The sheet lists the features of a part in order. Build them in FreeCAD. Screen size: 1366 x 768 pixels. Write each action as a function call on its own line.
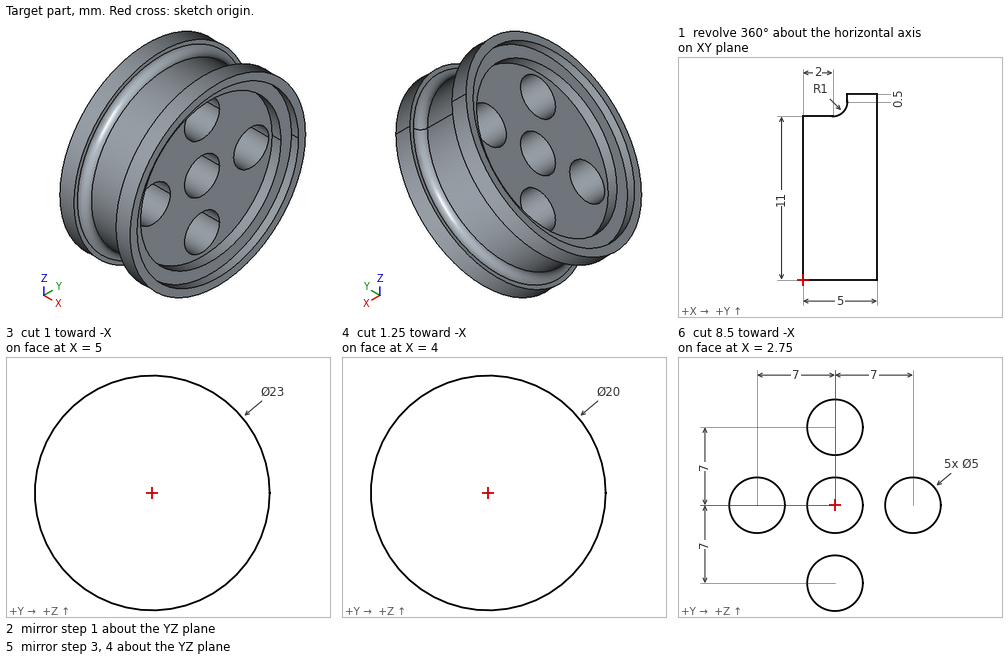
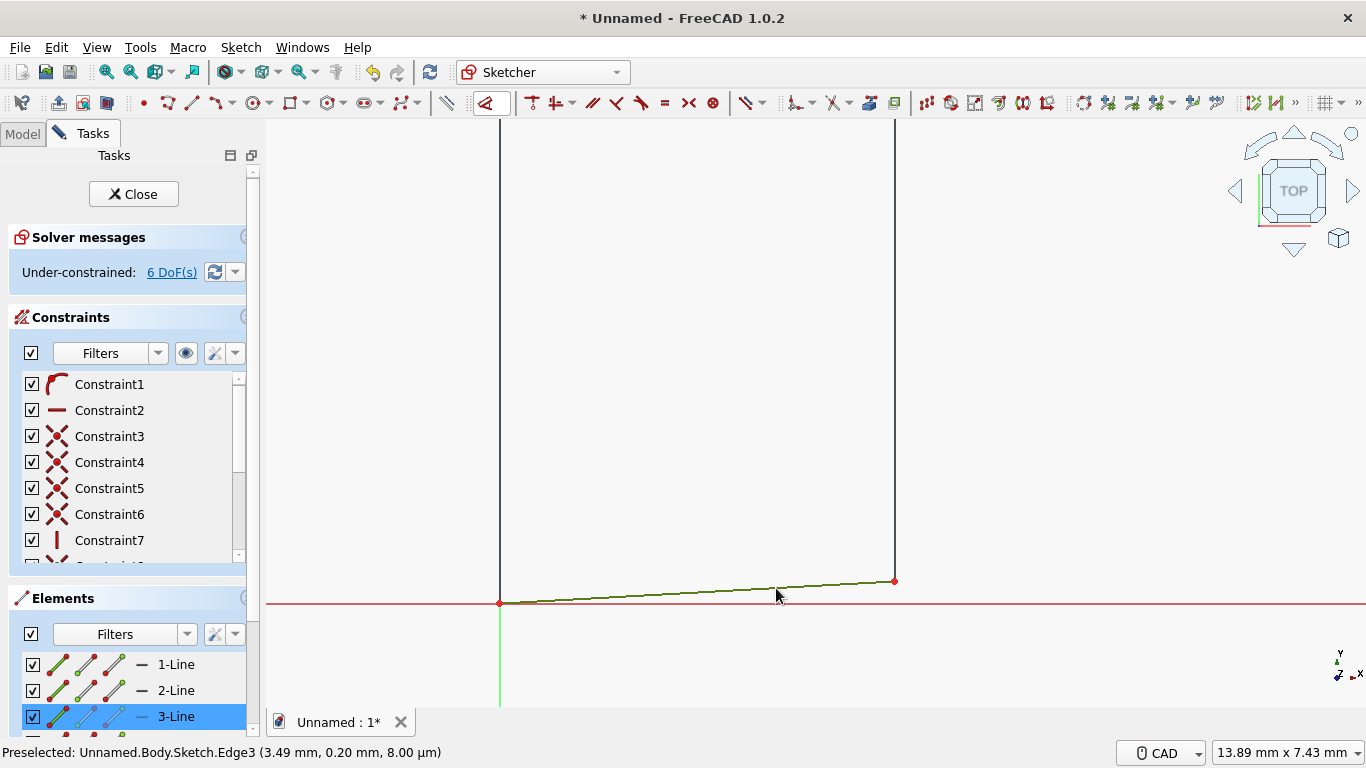
key(h)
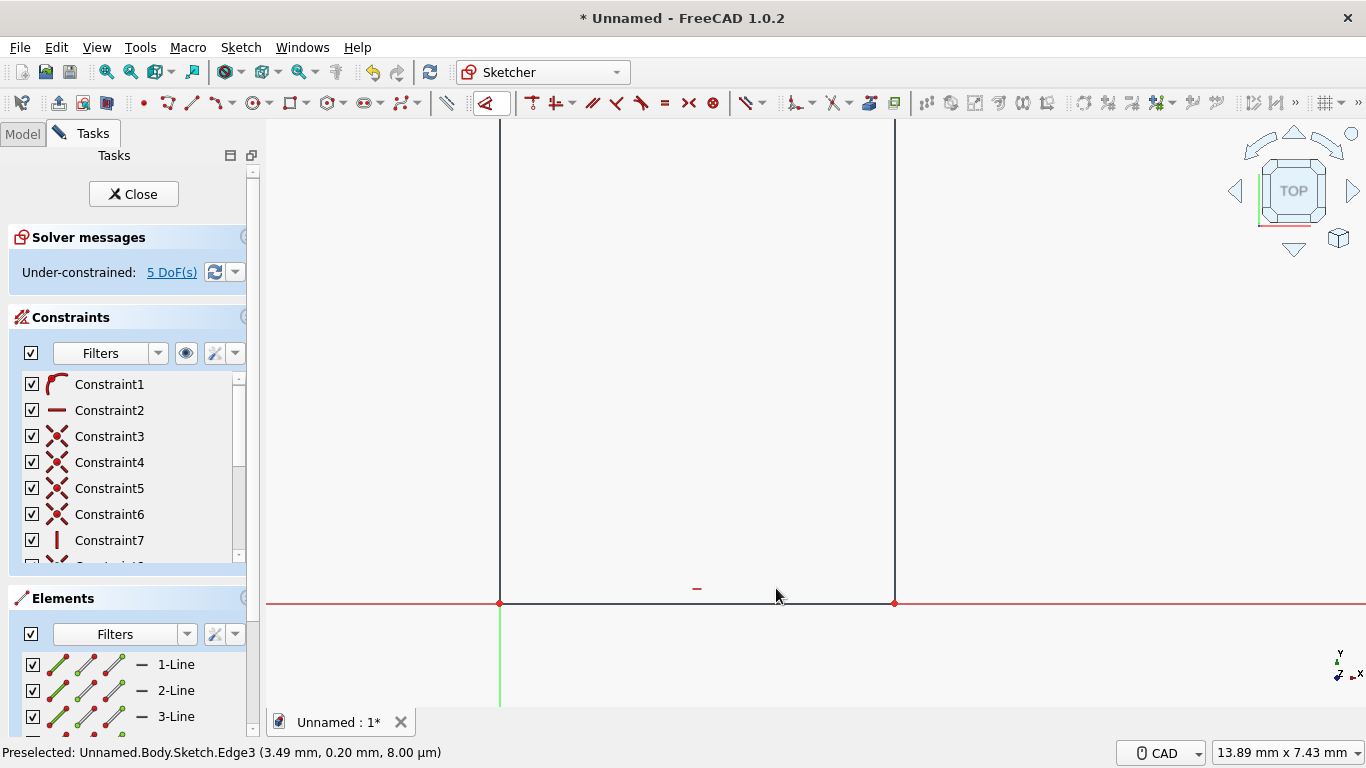
key(d)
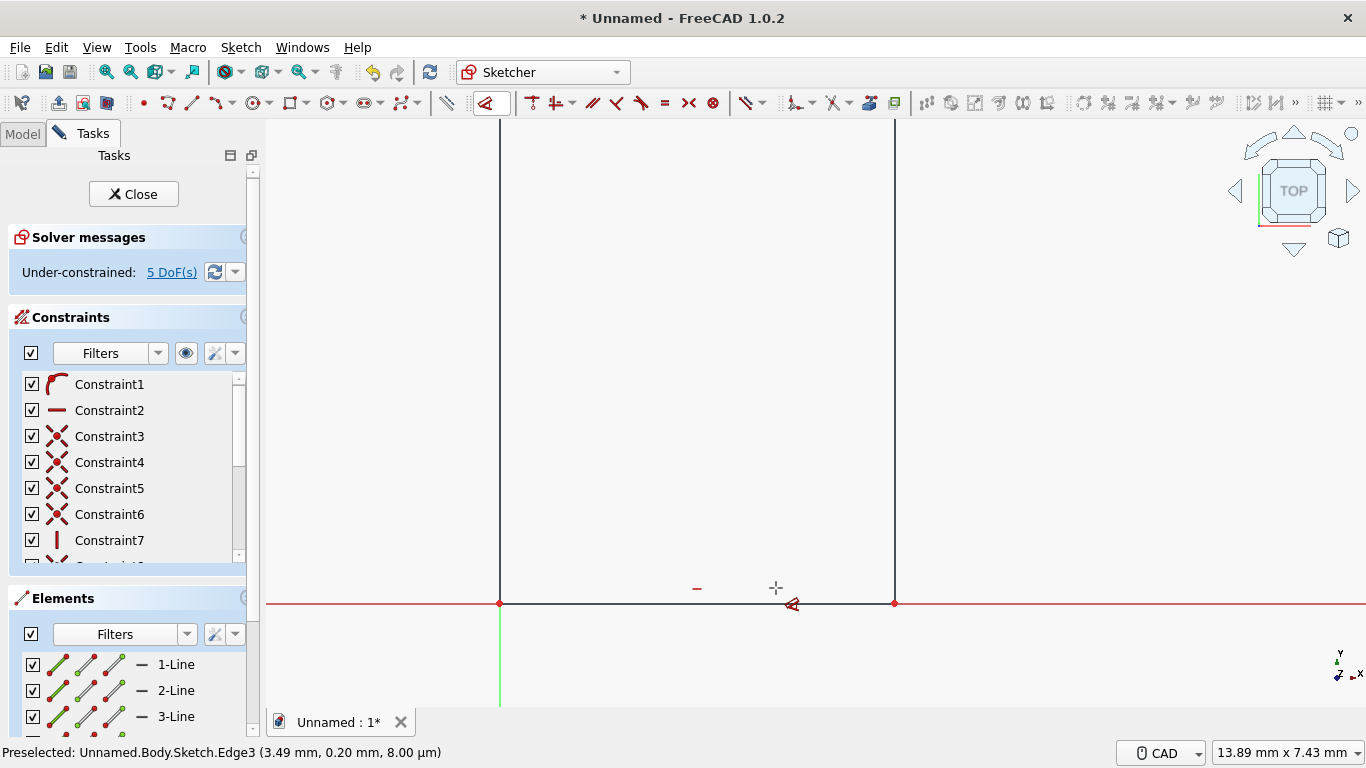
scroll(777, 590, down, 5)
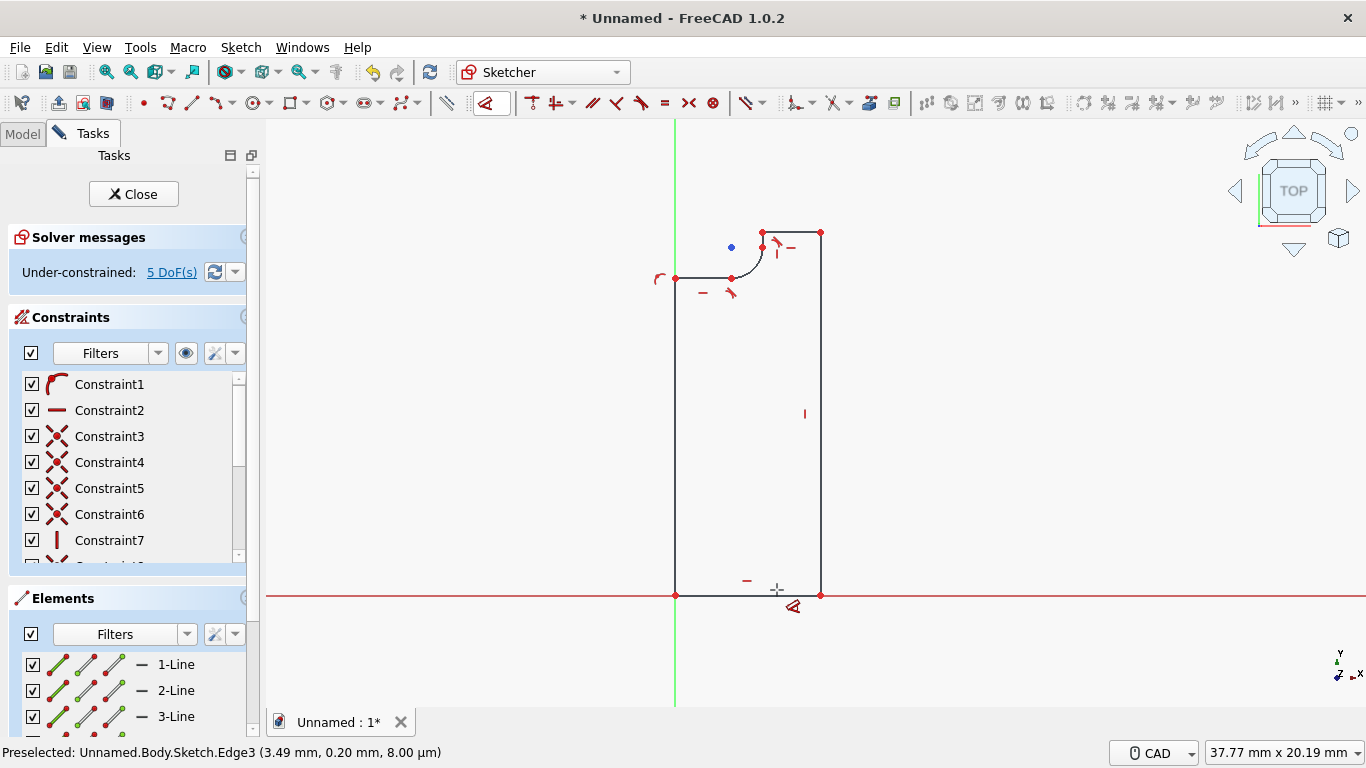
scroll(746, 275, up, 2)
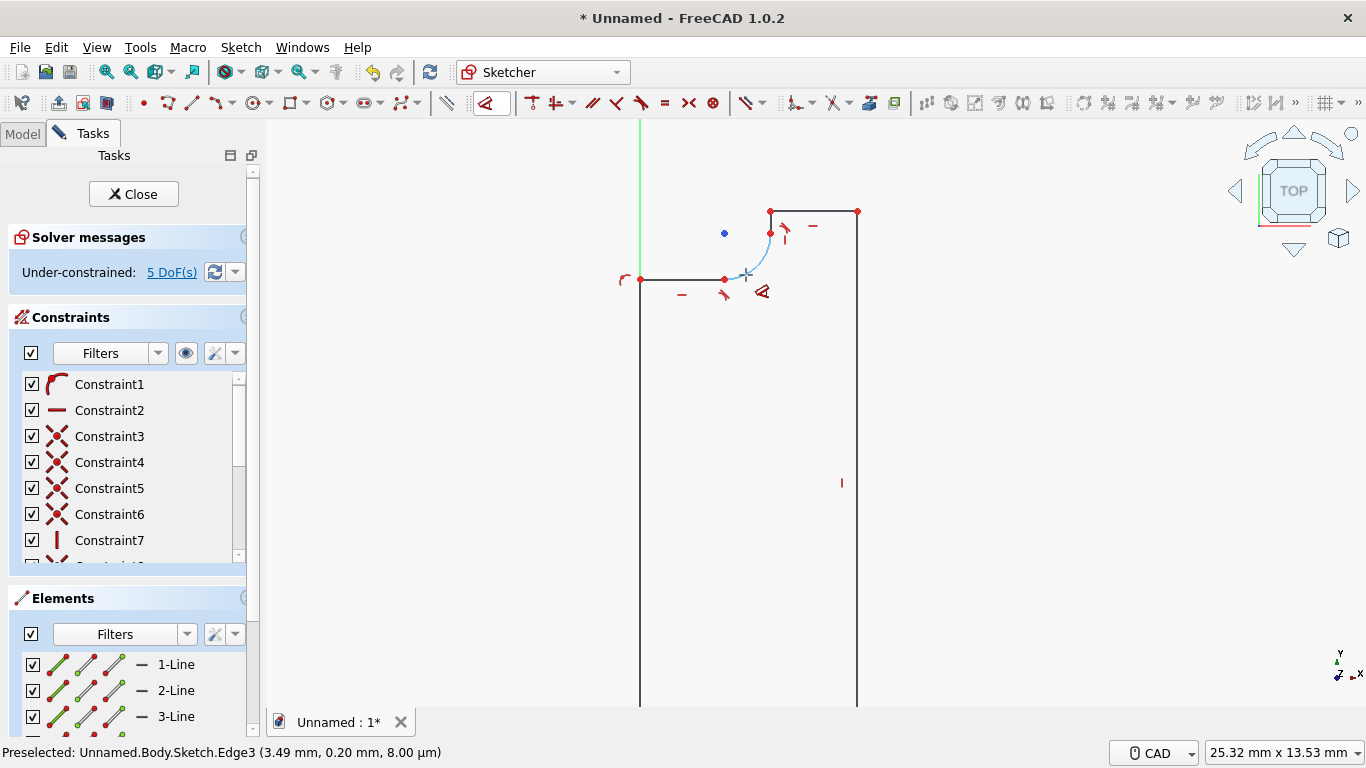
click(746, 275)
click(761, 303)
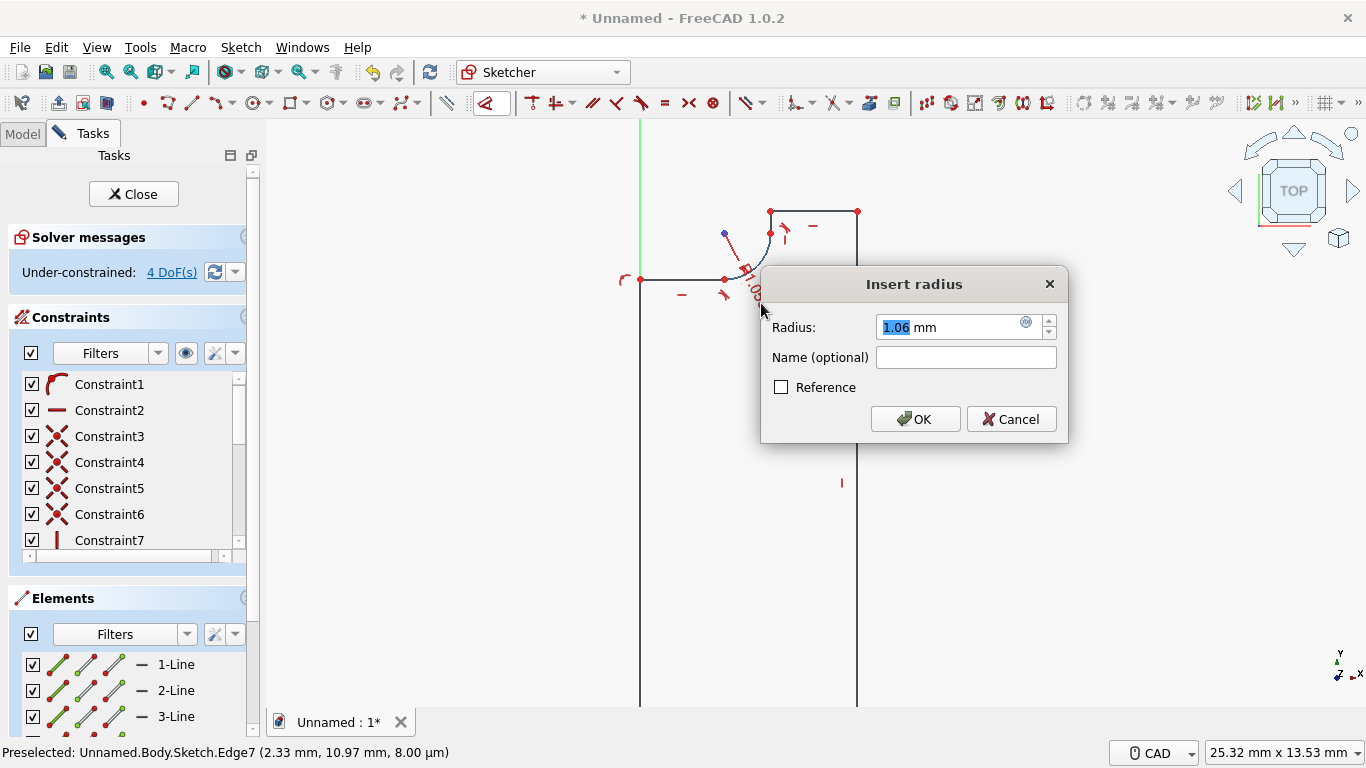
text(1)
key(Return)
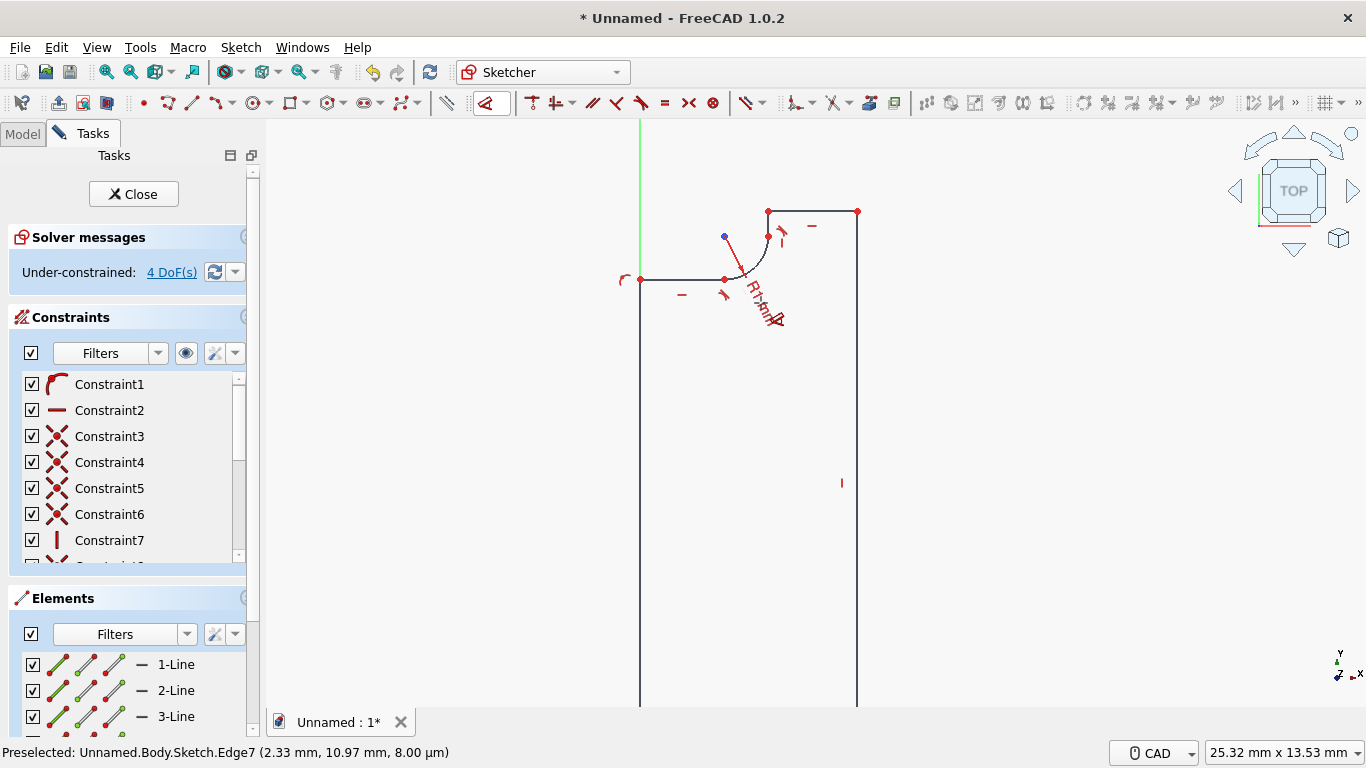
click(699, 280)
click(682, 246)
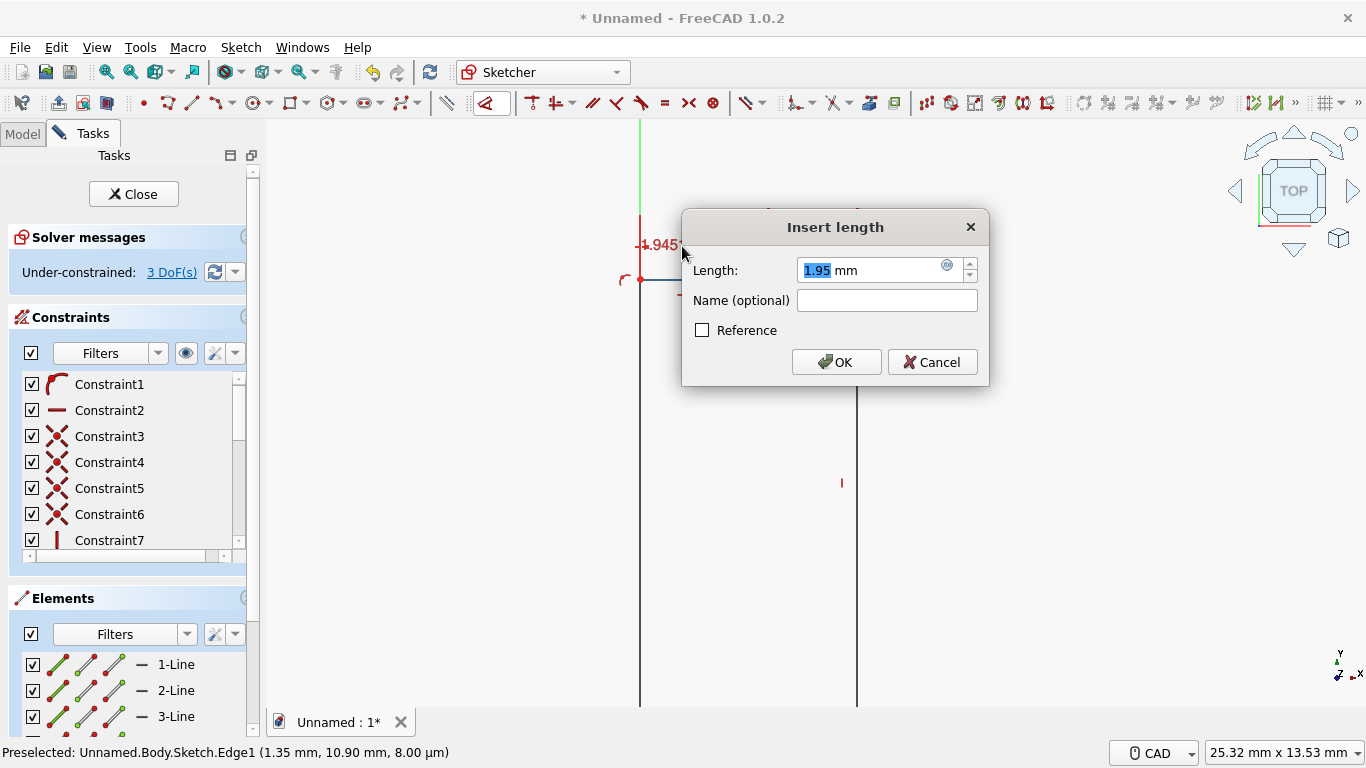
text(2)
key(Return)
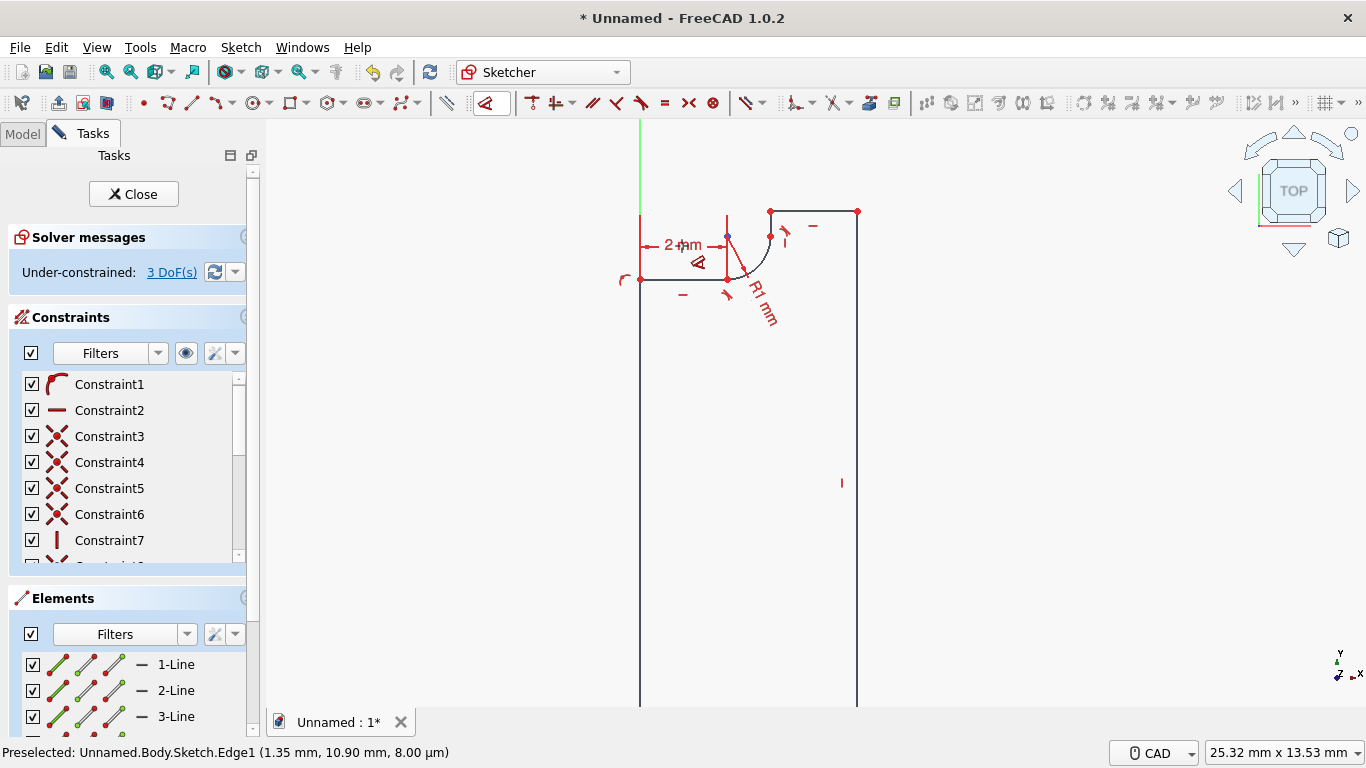
scroll(745, 274, down, 2)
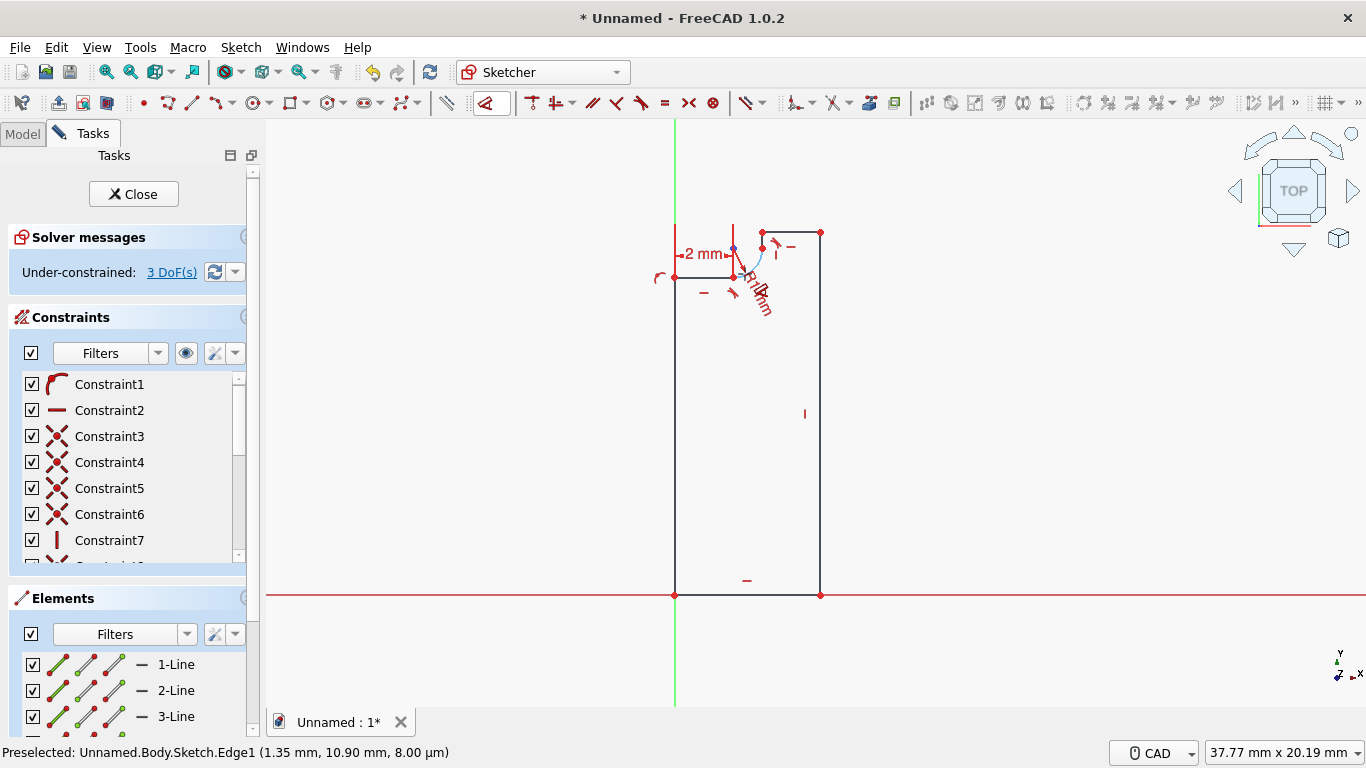
click(719, 595)
click(748, 629)